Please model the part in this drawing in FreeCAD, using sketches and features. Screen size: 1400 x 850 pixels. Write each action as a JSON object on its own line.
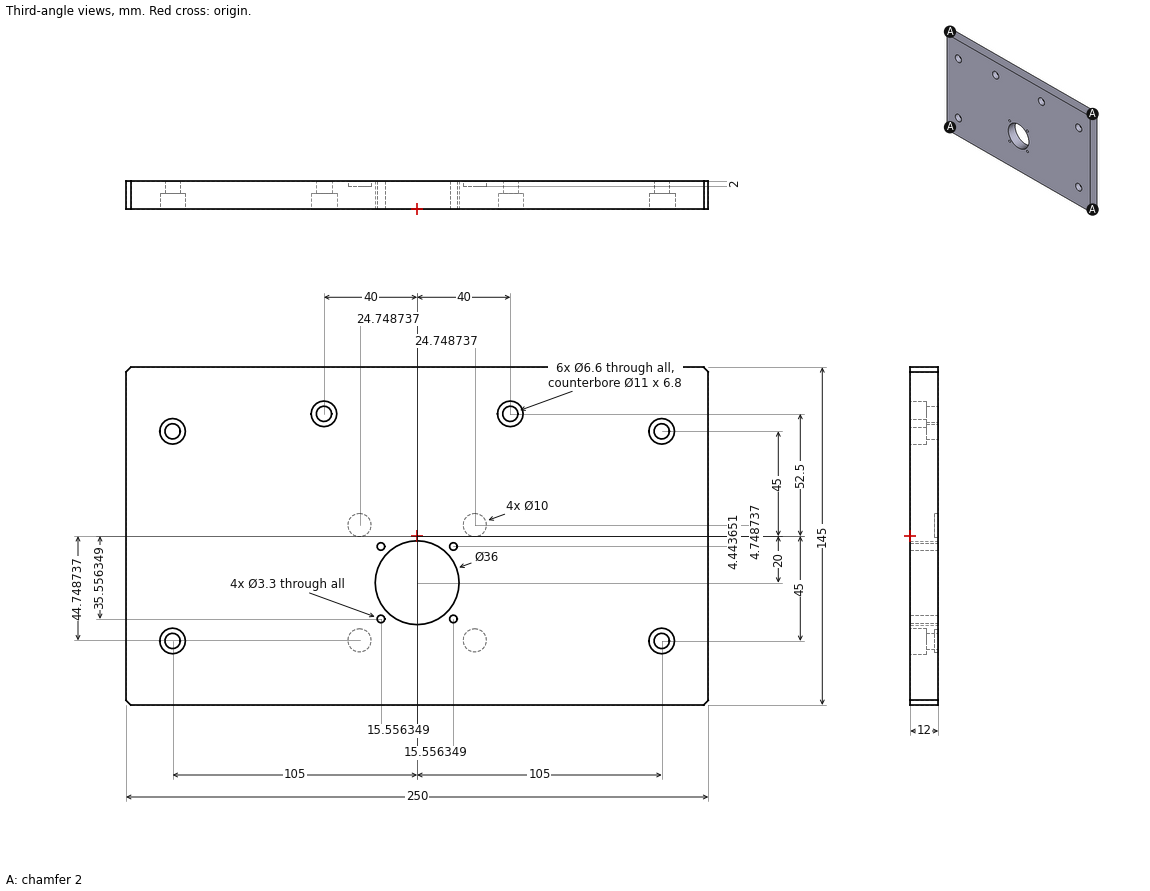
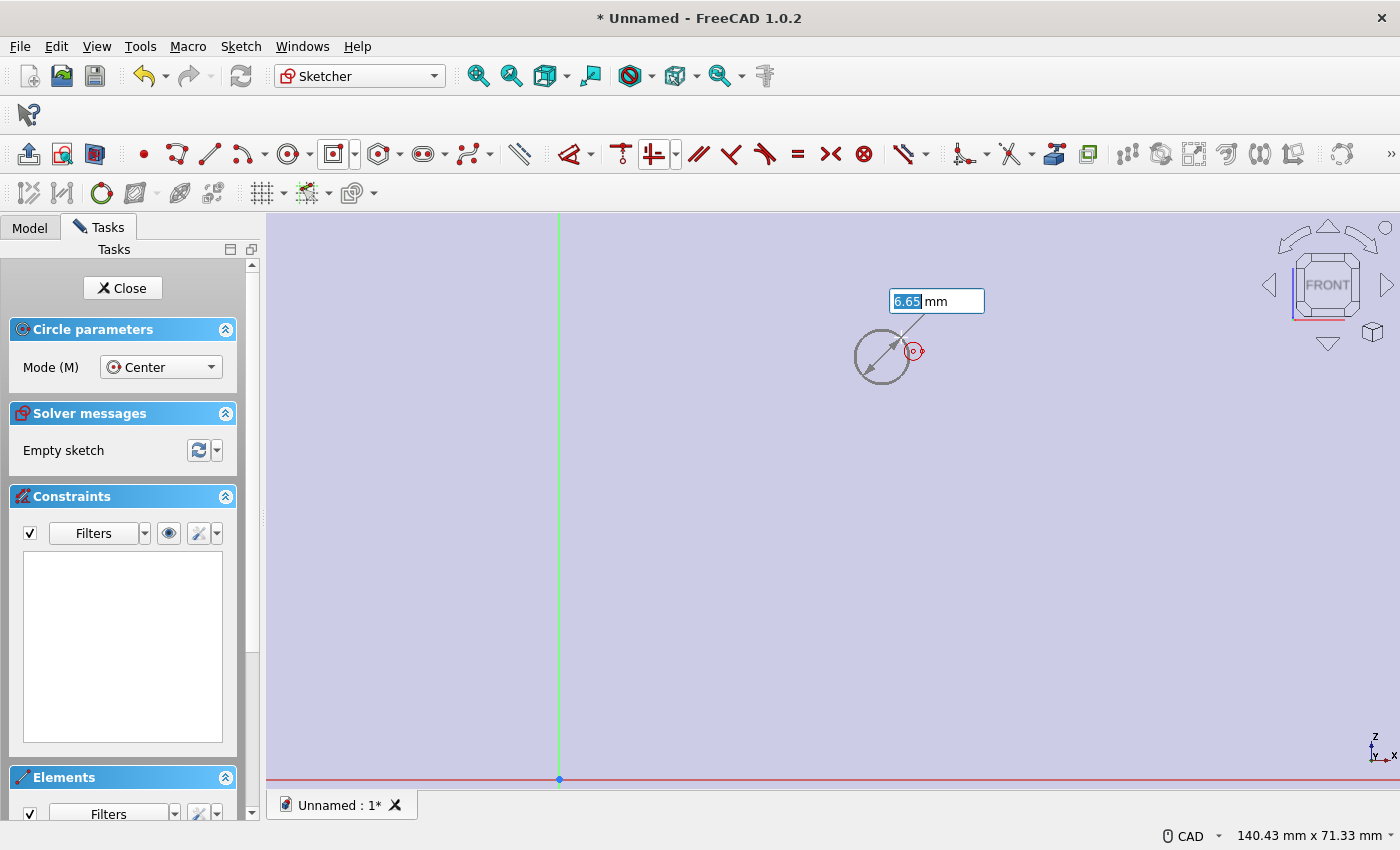
{"action": "type", "text": "6.6"}
{"action": "key", "text": "Return"}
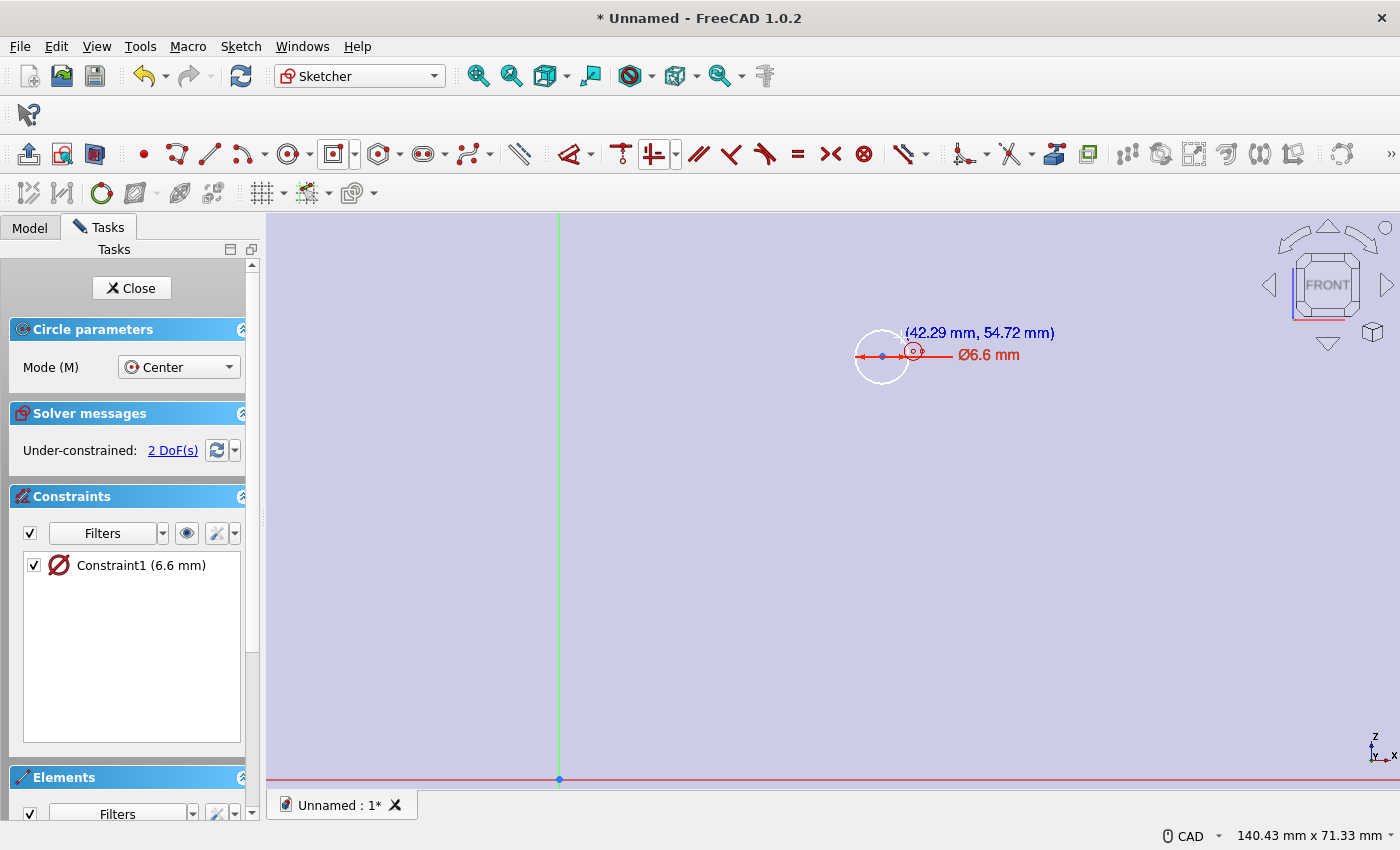
{"action": "scroll", "coordinate": [884, 356], "scroll_direction": "down", "scroll_amount": 5}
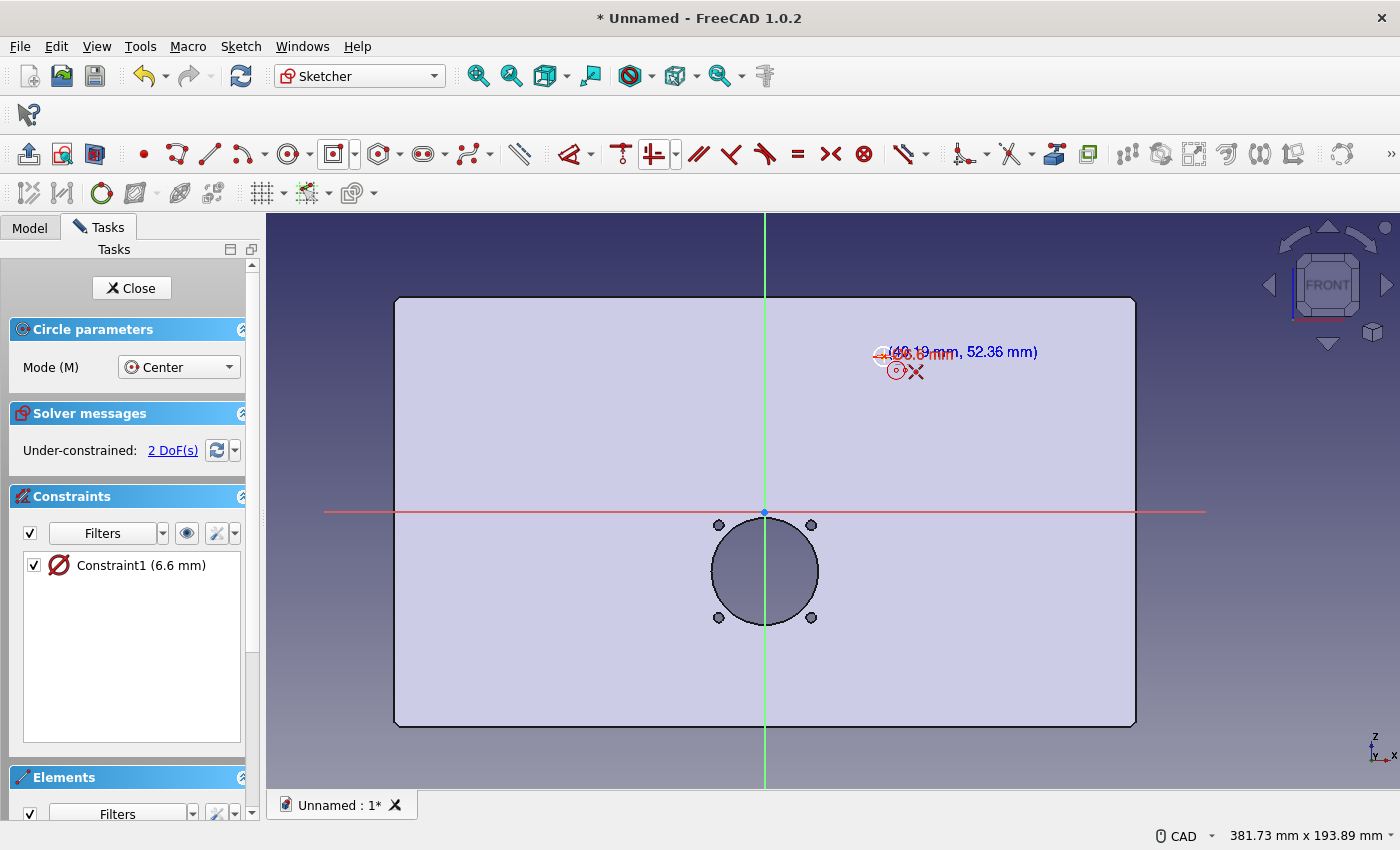
{"action": "scroll", "coordinate": [1077, 646], "scroll_direction": "up", "scroll_amount": 5}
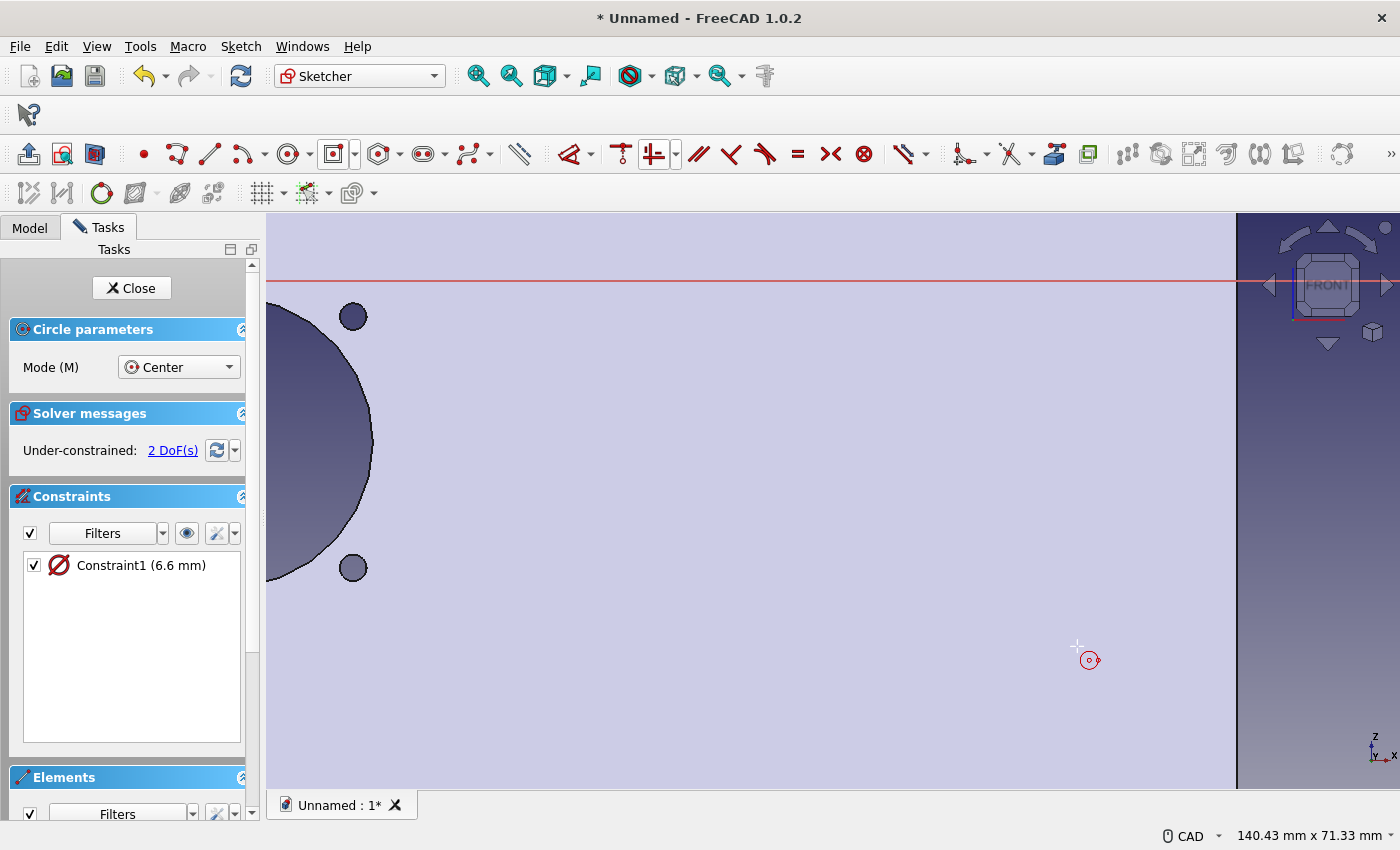
{"action": "left_click", "coordinate": [1075, 644]}
{"action": "mouse_move", "coordinate": [1094, 625]}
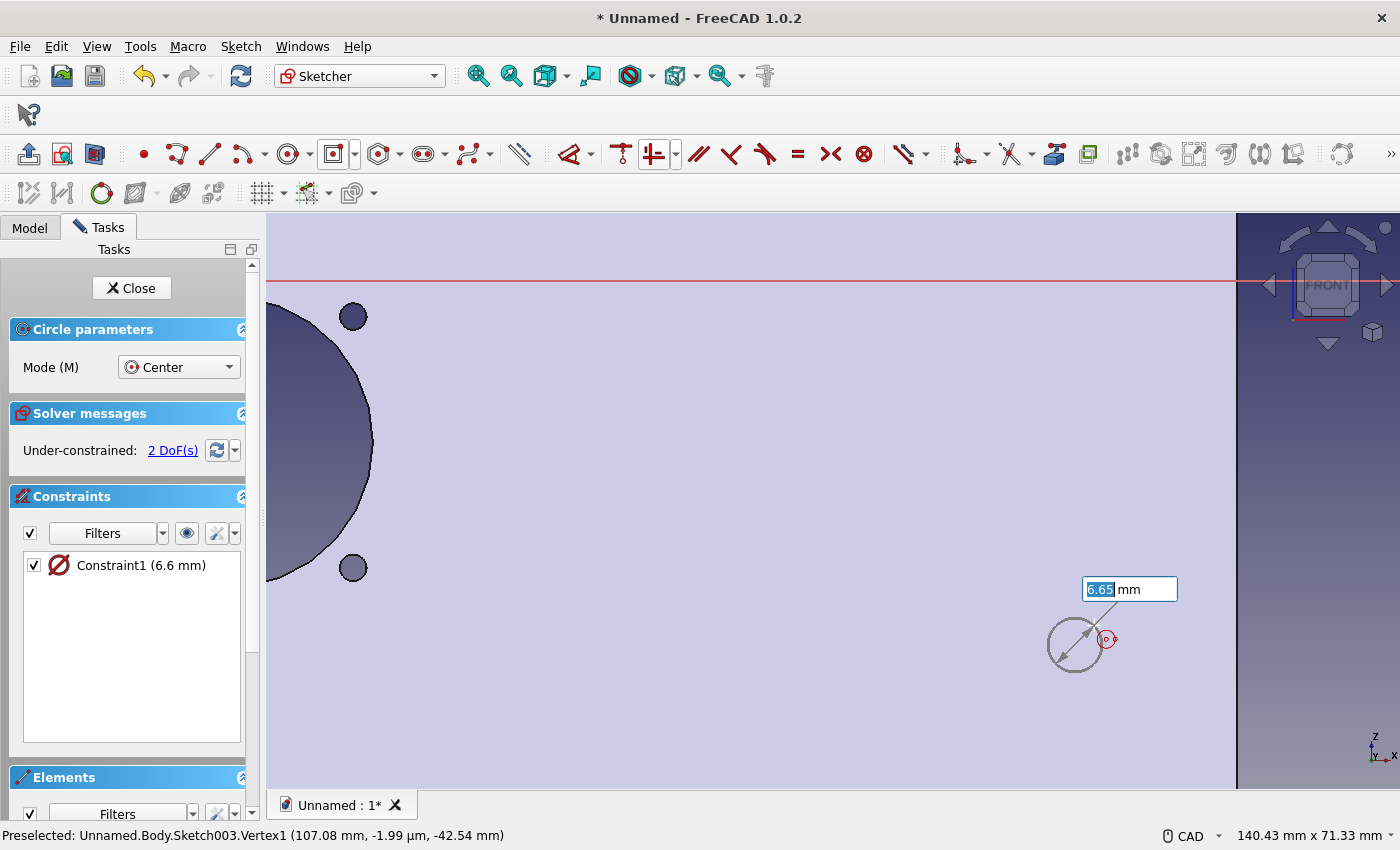
{"action": "type", "text": "6.6"}
{"action": "key", "text": "Return"}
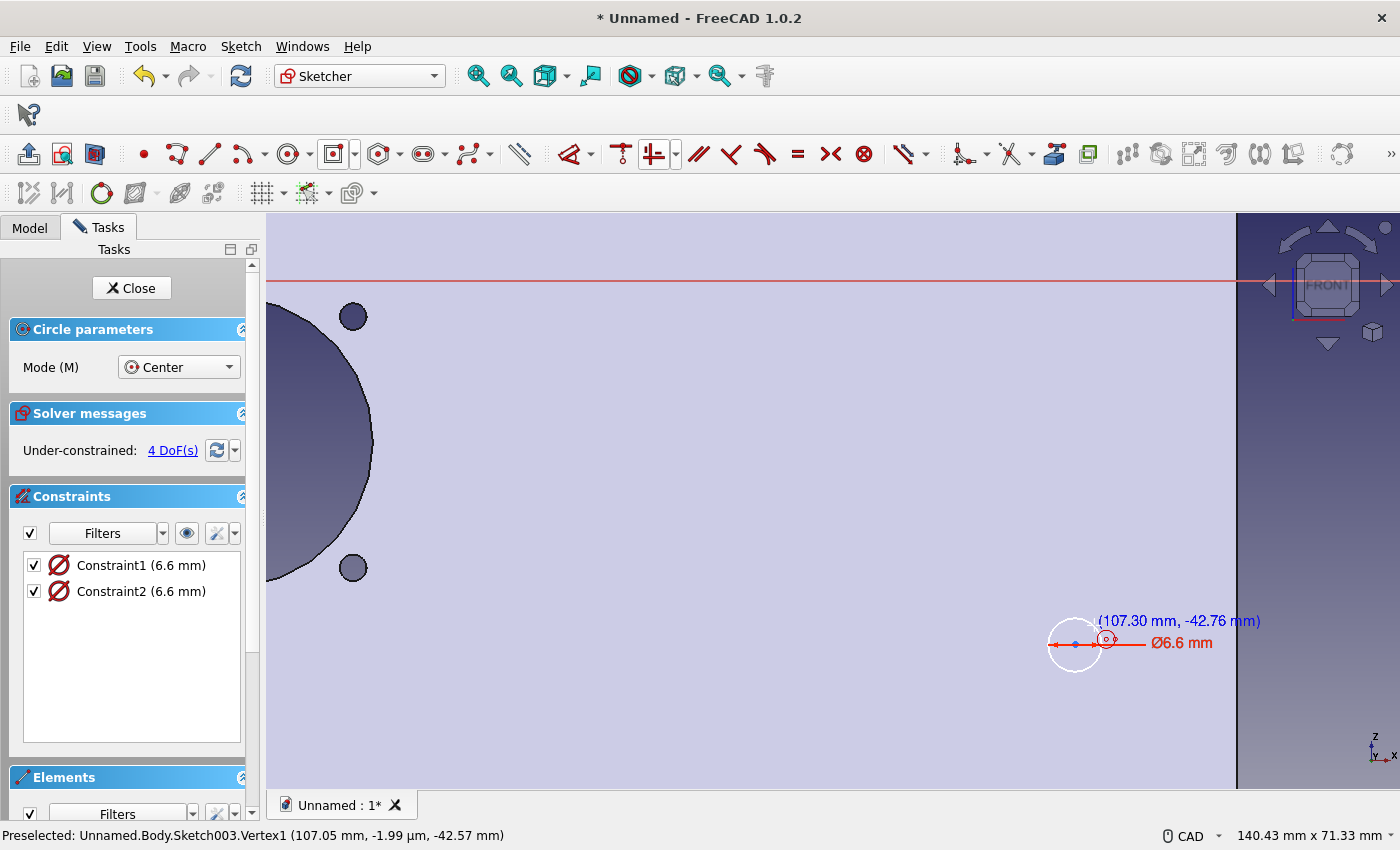
{"action": "scroll", "coordinate": [1077, 647], "scroll_direction": "down", "scroll_amount": 5}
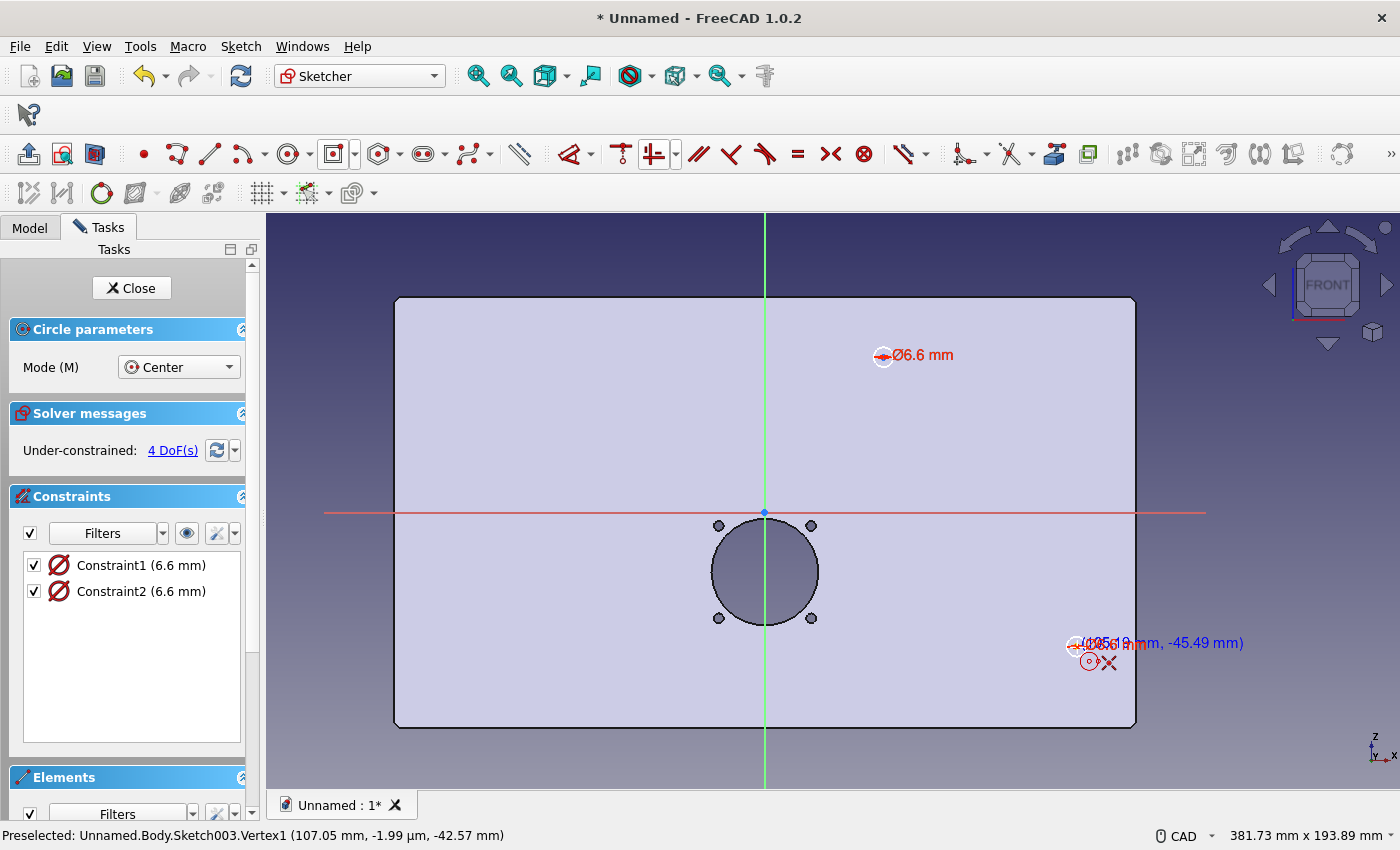
{"action": "scroll", "coordinate": [1077, 379], "scroll_direction": "up", "scroll_amount": 5}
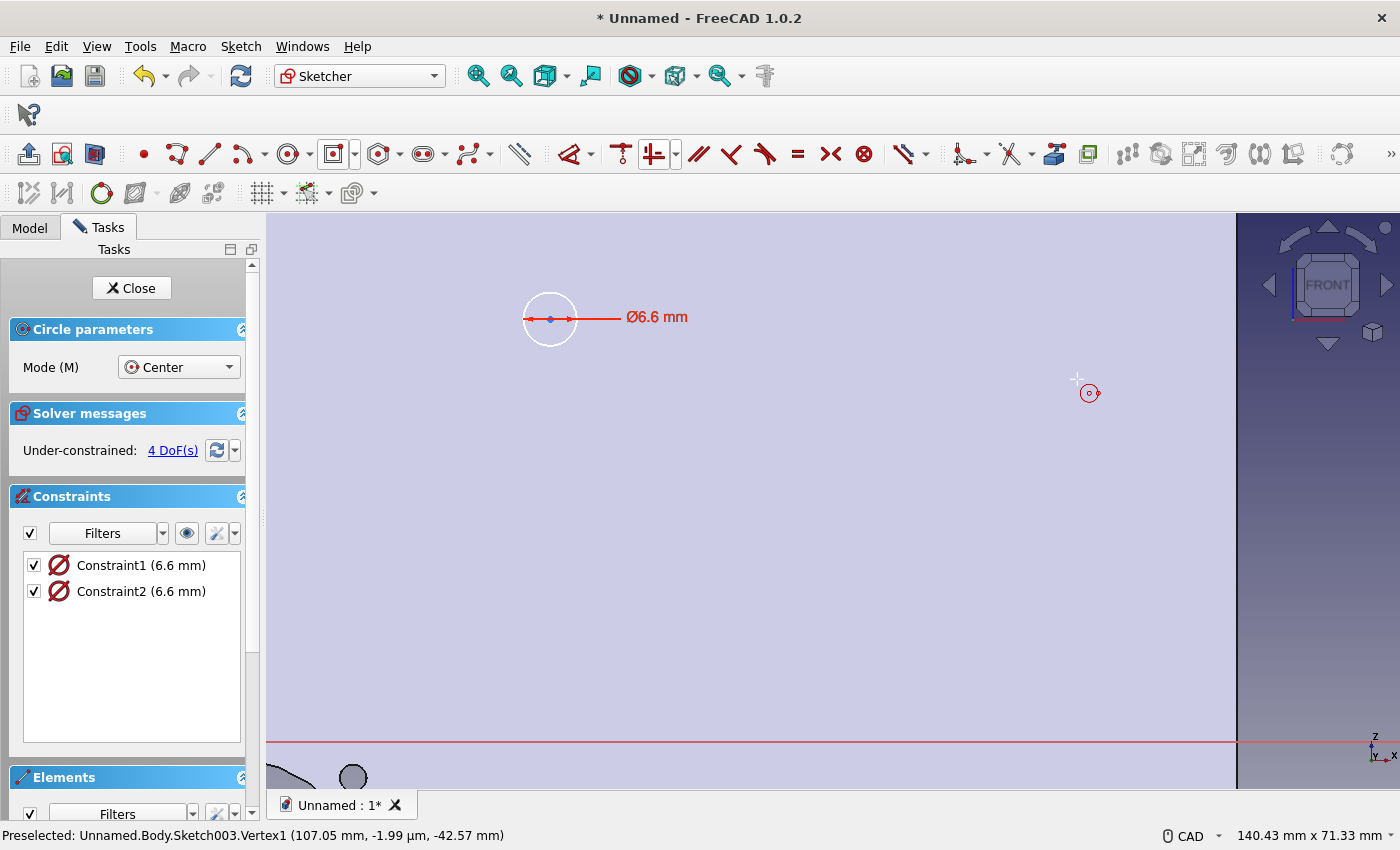
{"action": "left_click", "coordinate": [1075, 379]}
{"action": "mouse_move", "coordinate": [1094, 360]}